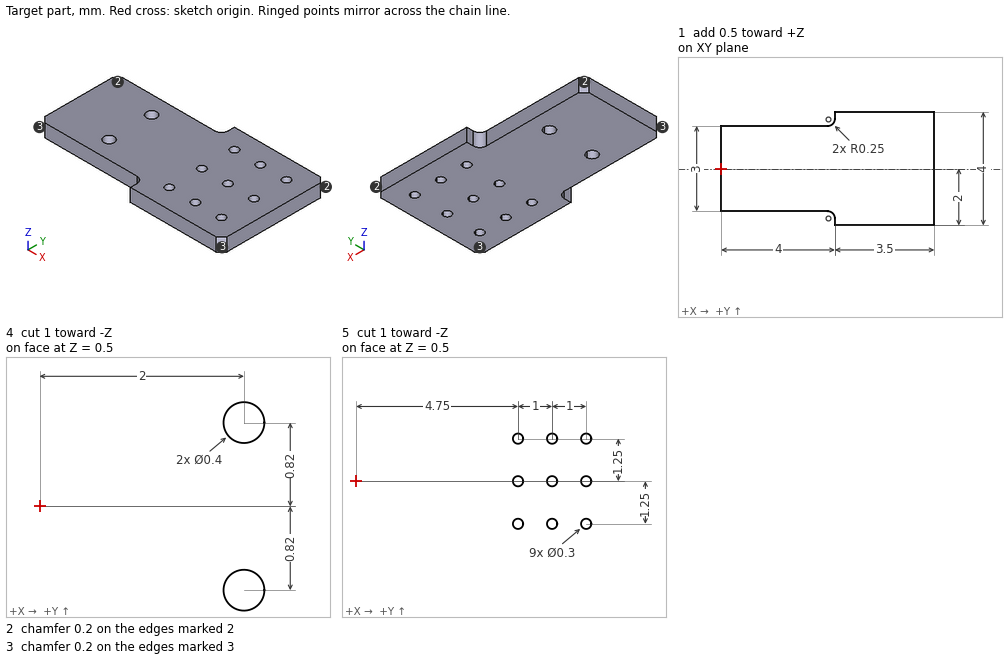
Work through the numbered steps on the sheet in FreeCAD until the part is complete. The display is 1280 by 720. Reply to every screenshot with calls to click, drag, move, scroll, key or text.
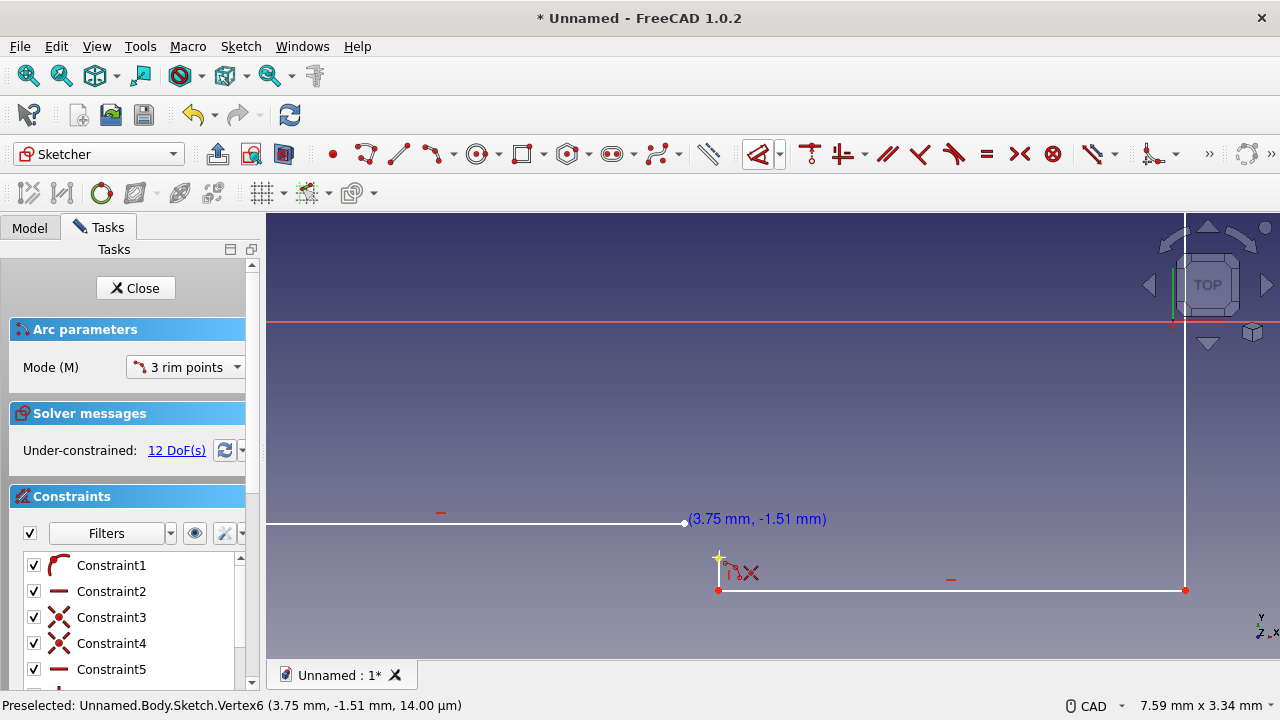
click(719, 558)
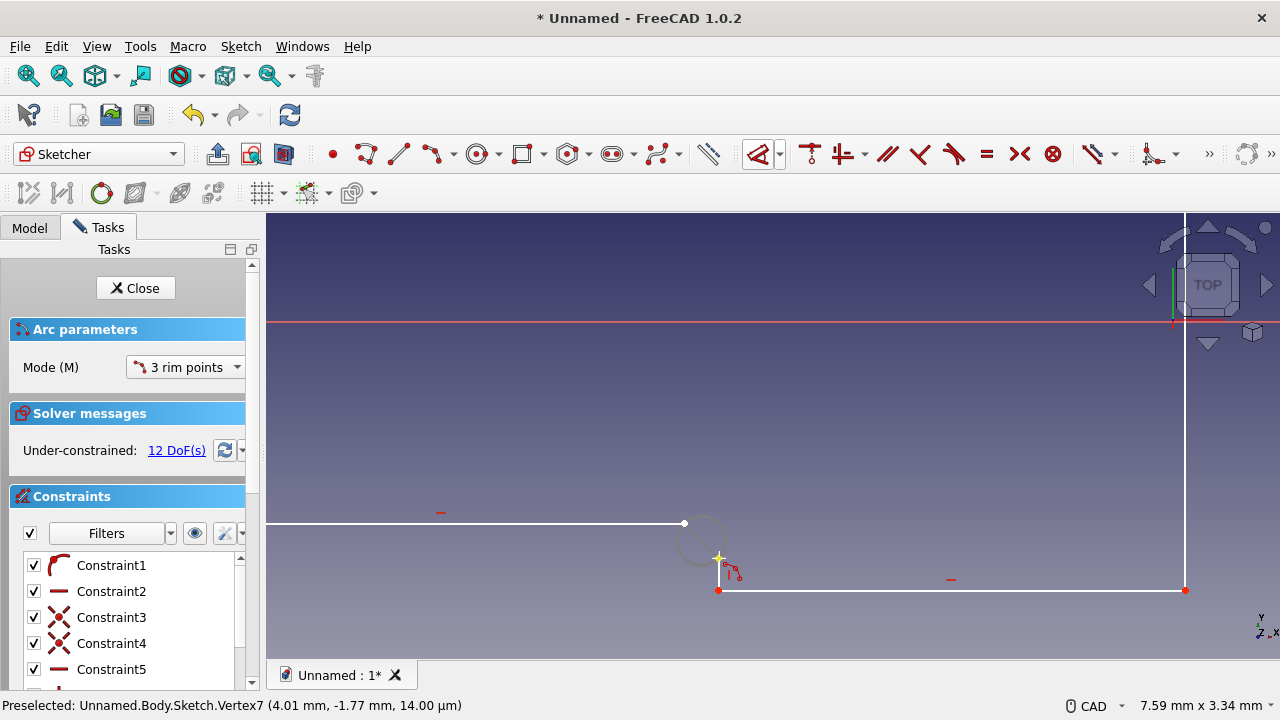
scroll(708, 532, up, 3)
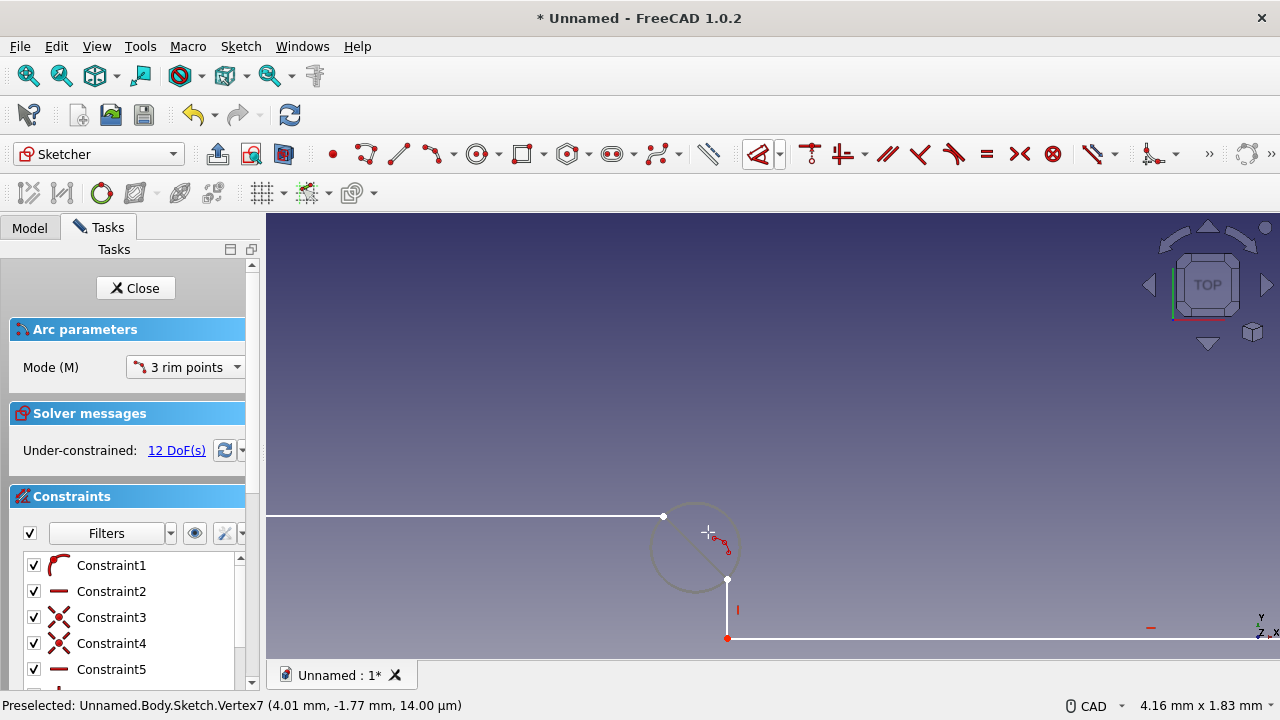
click(708, 531)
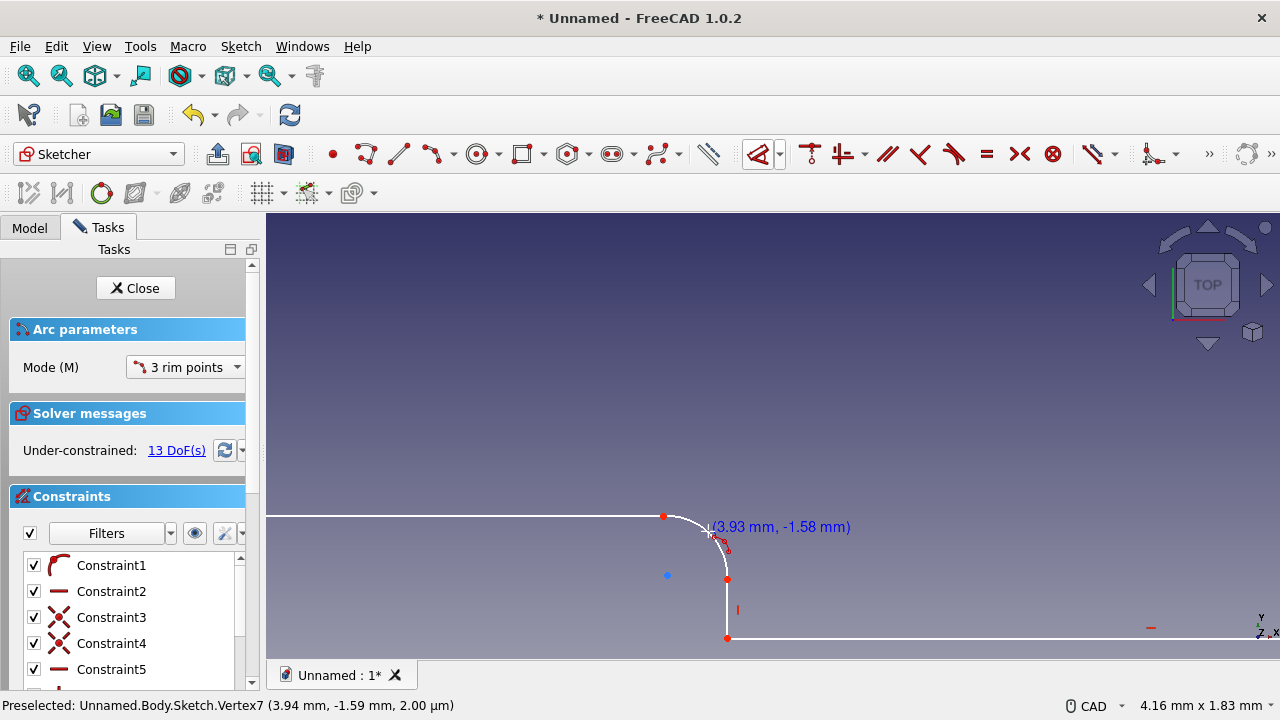
scroll(722, 560, down, 6)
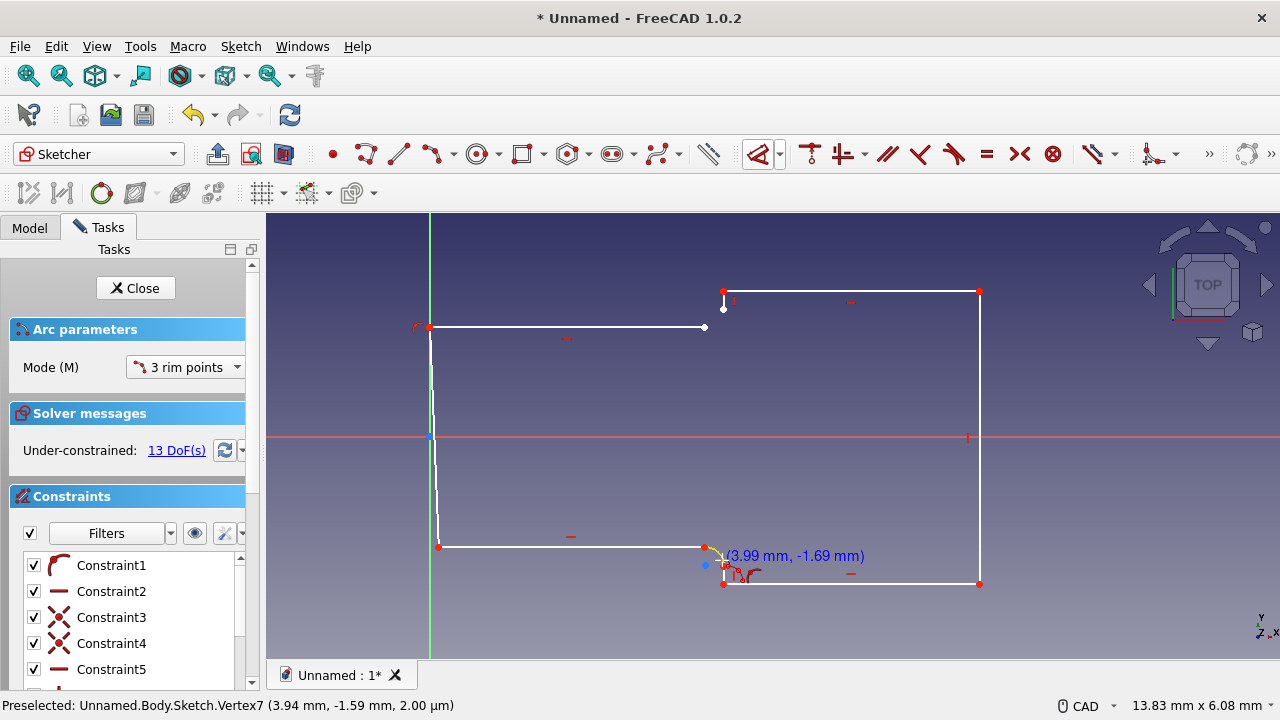
scroll(723, 308, up, 3)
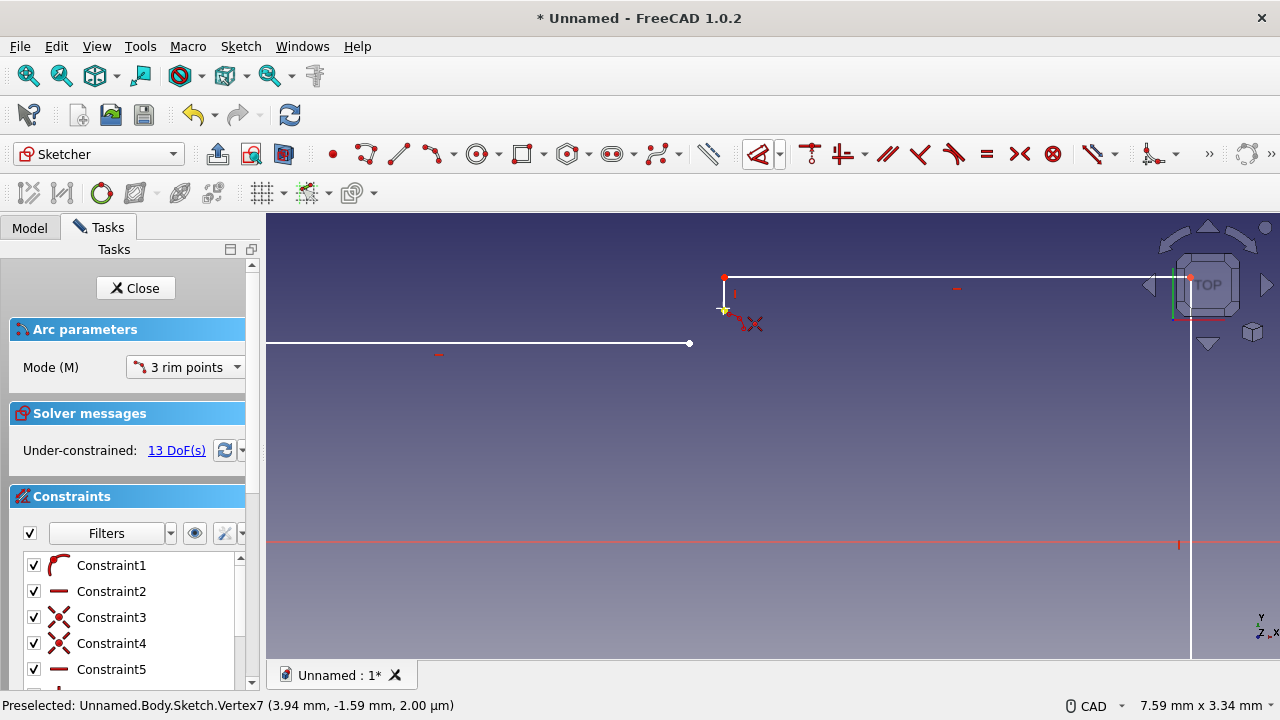
click(724, 310)
click(690, 343)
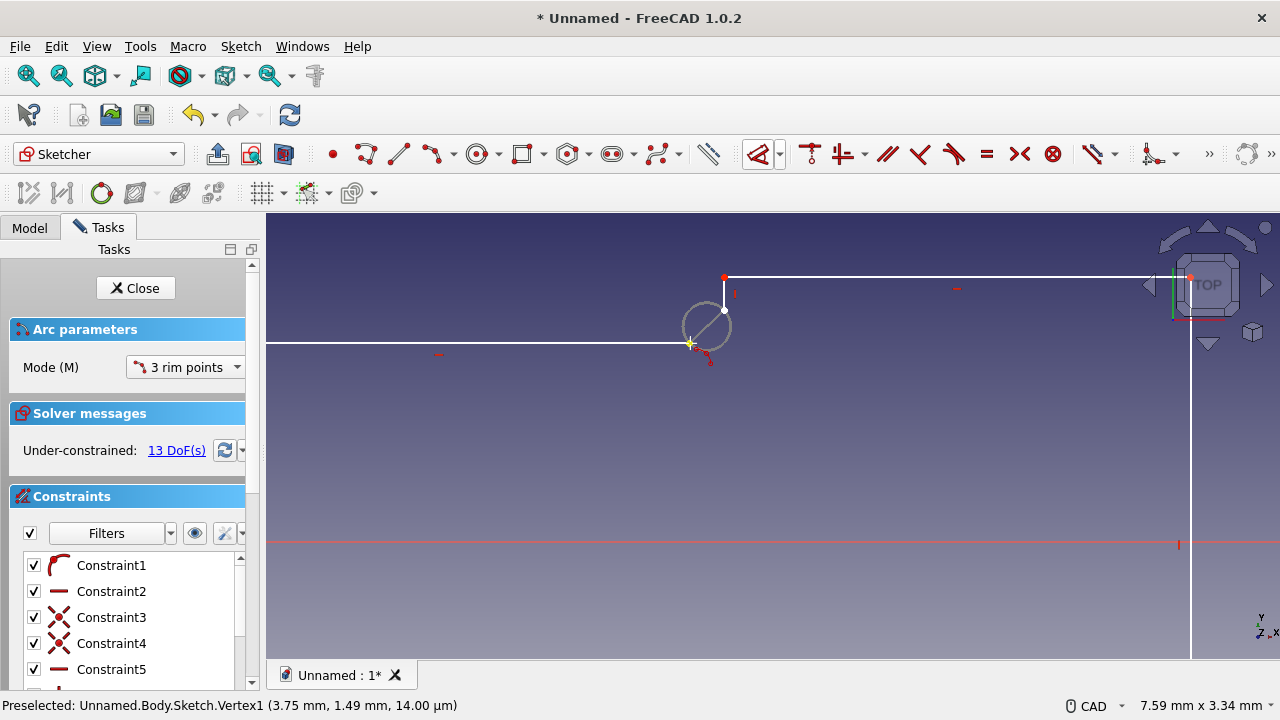
scroll(713, 332, up, 3)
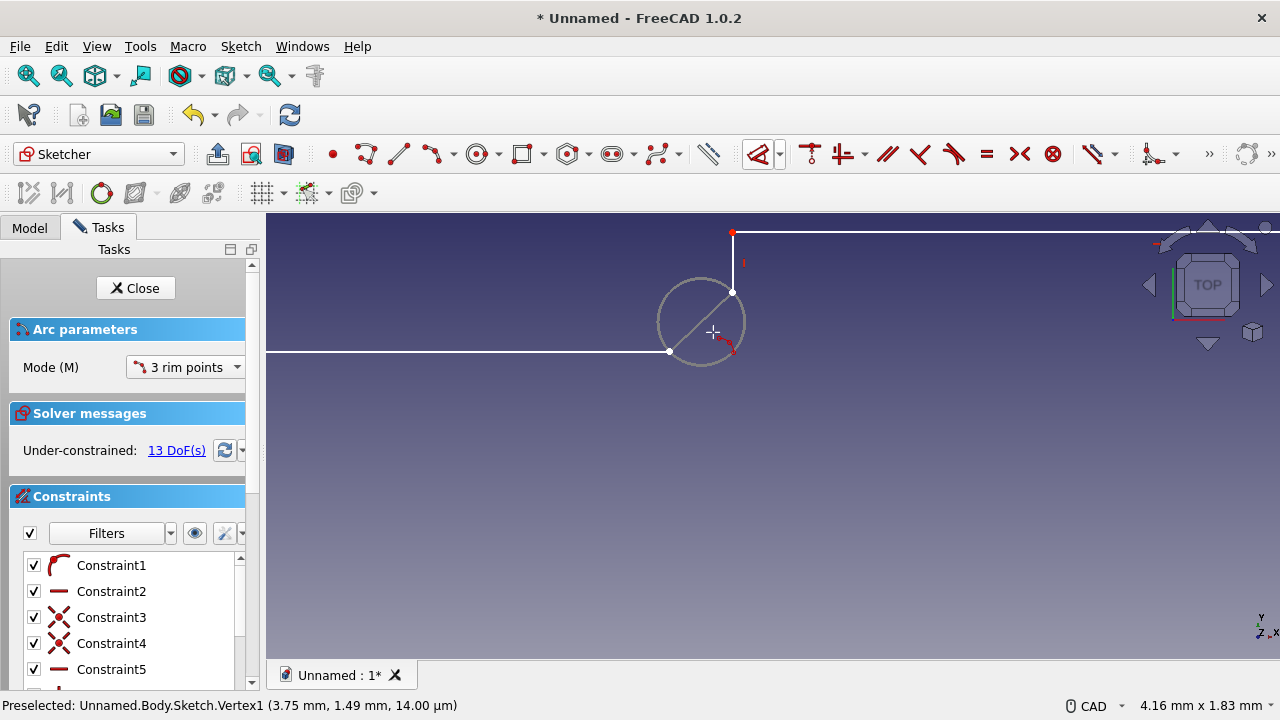
click(714, 331)
key(Escape)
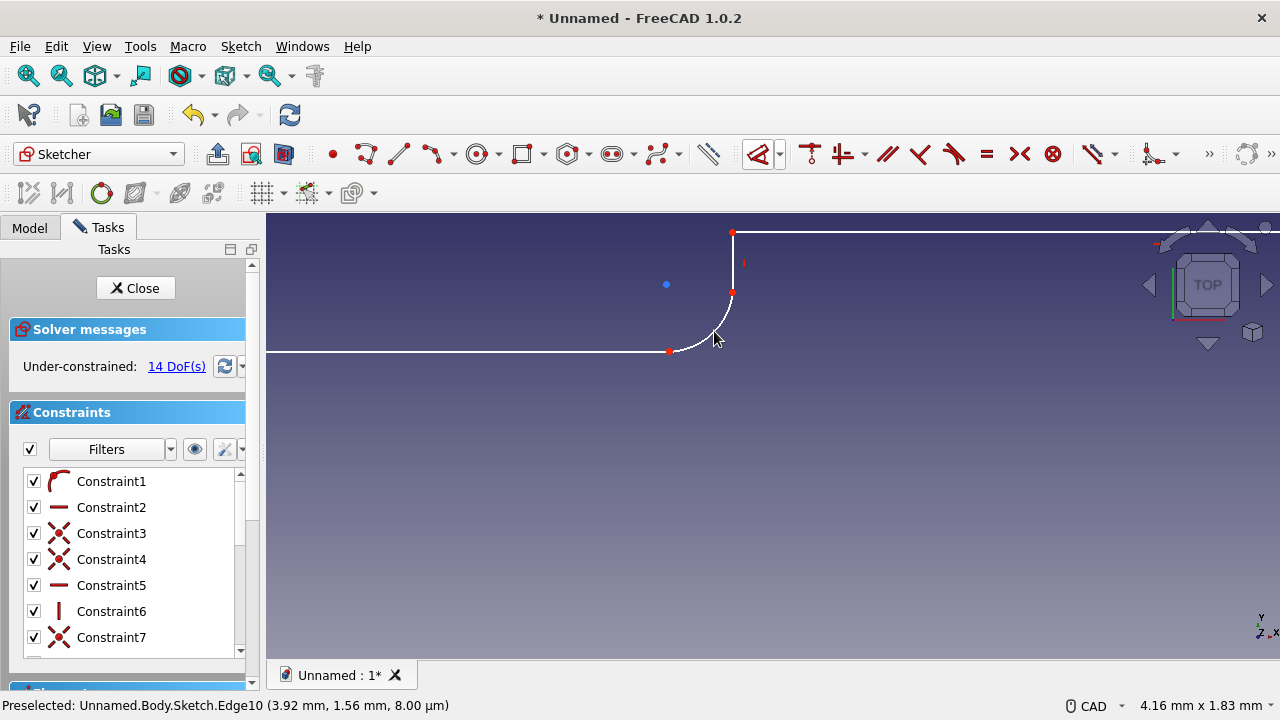
click(396, 352)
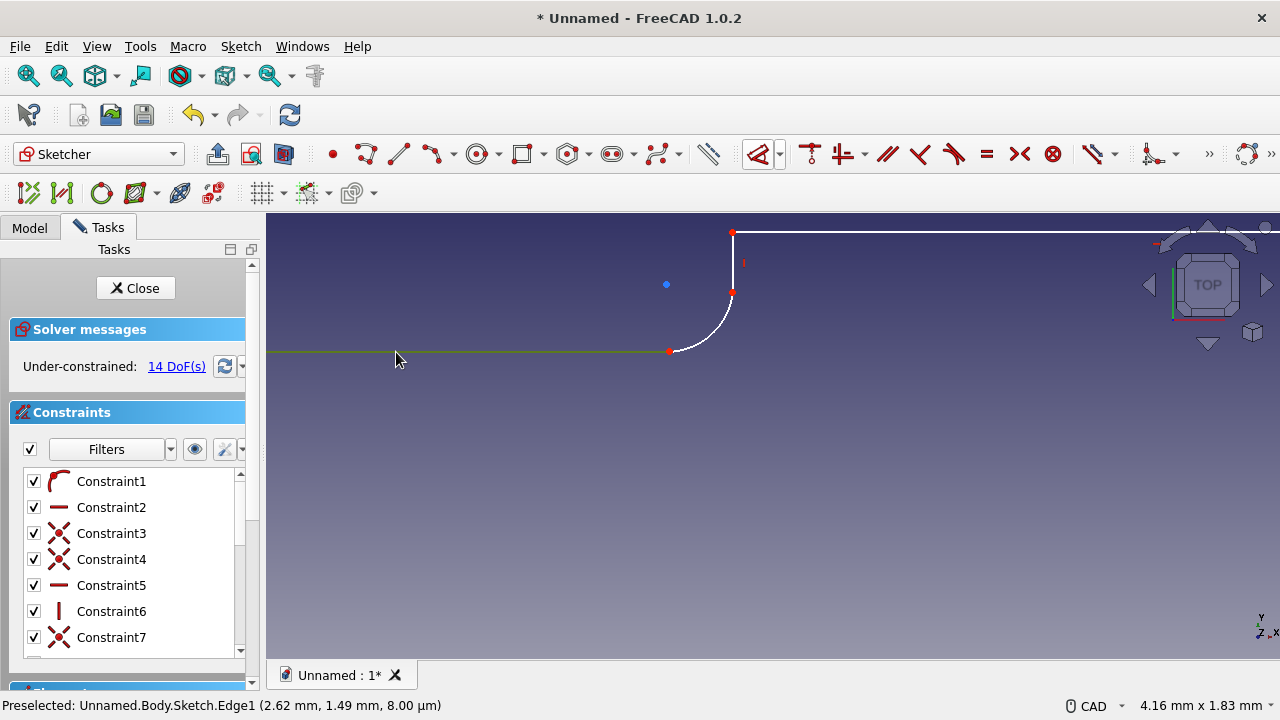
click(697, 344)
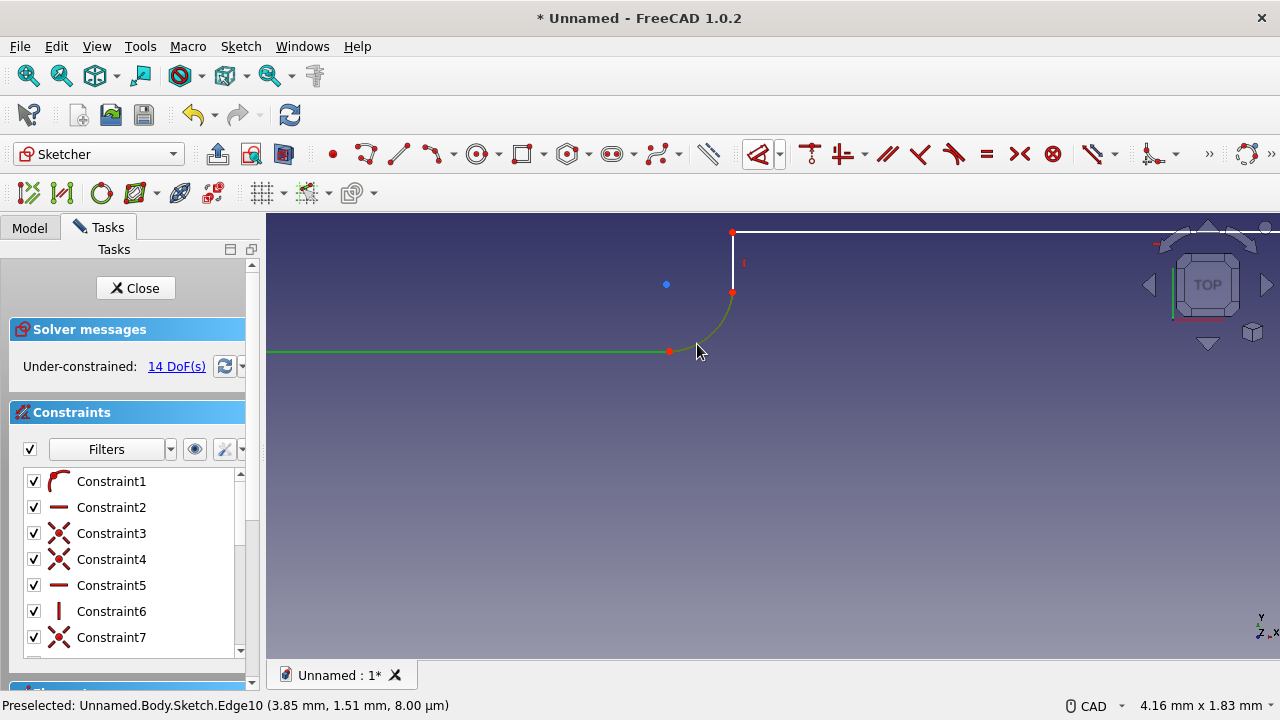
key(t)